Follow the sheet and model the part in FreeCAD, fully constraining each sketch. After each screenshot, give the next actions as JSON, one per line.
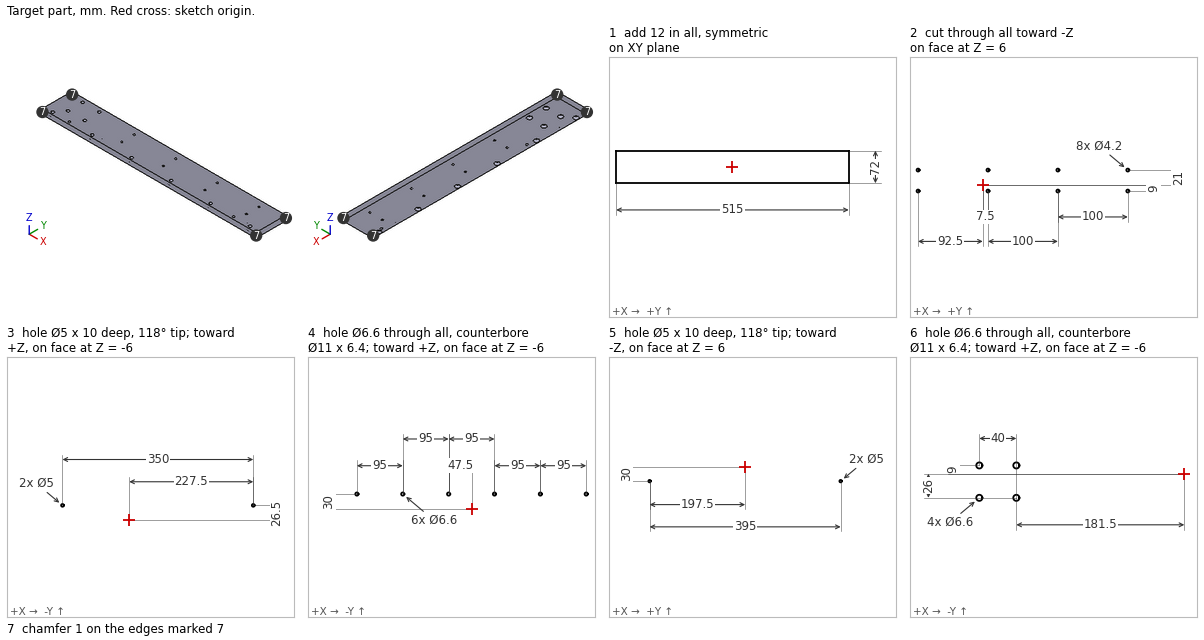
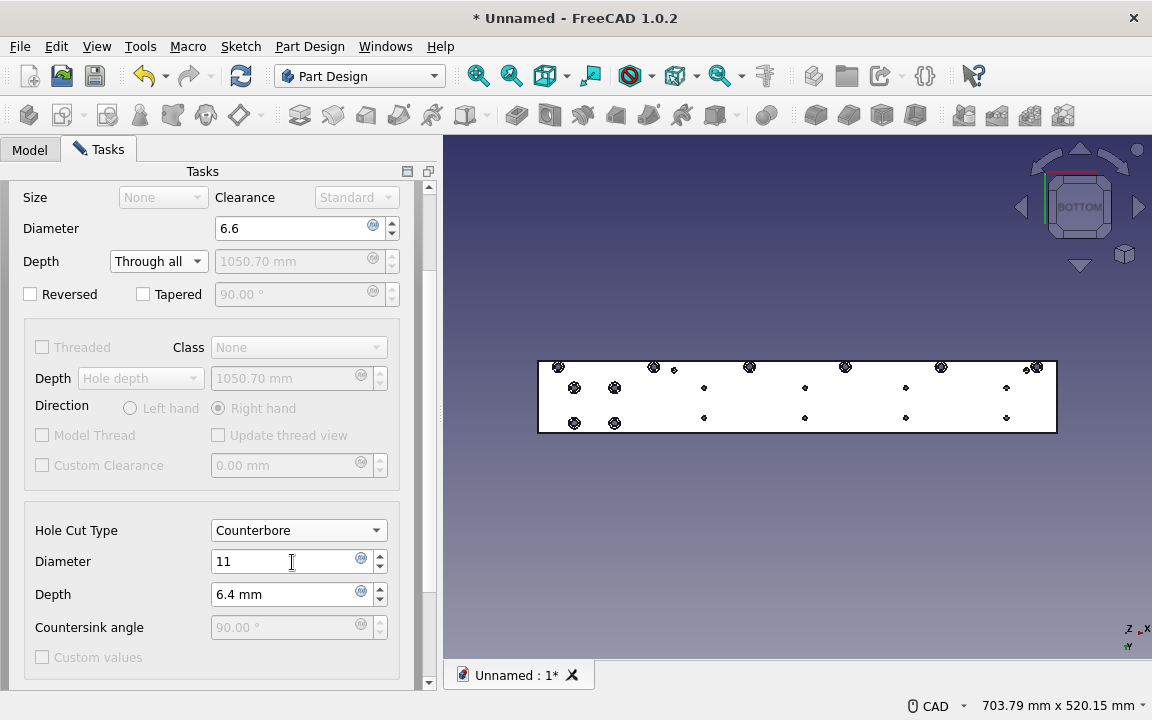
{"action": "scroll", "coordinate": [429, 436], "scroll_direction": "up", "scroll_amount": 3}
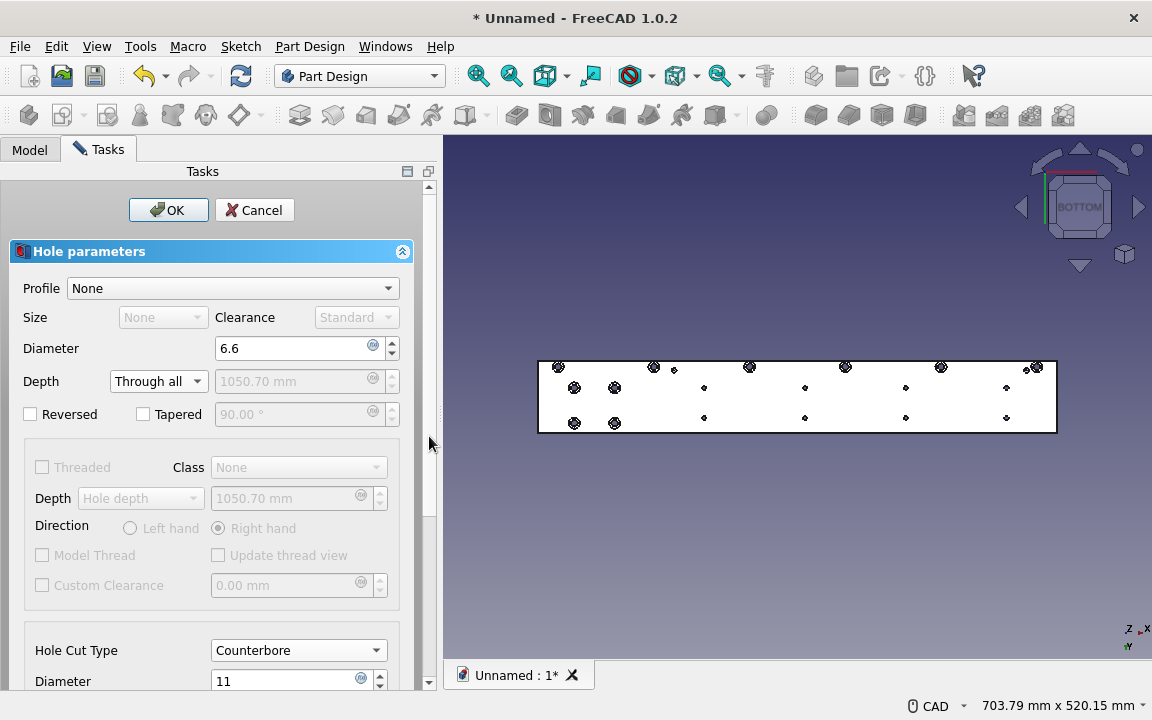
{"action": "left_click", "coordinate": [169, 210]}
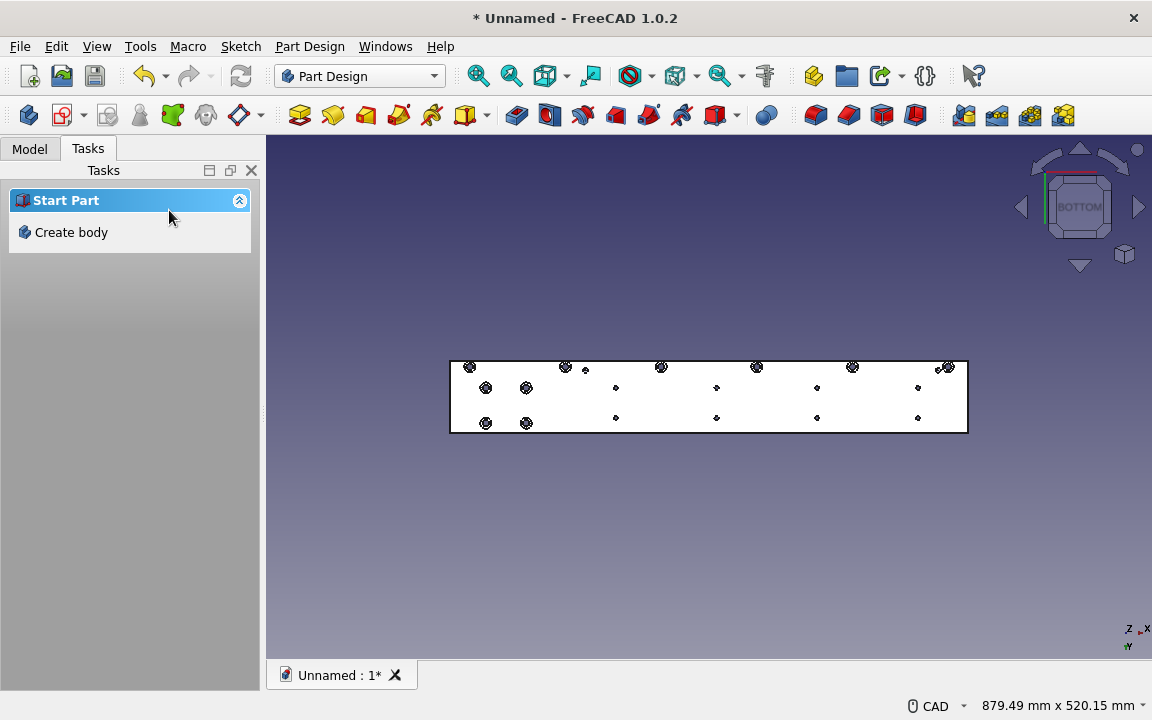
{"action": "scroll", "coordinate": [968, 360], "scroll_direction": "up", "scroll_amount": 6}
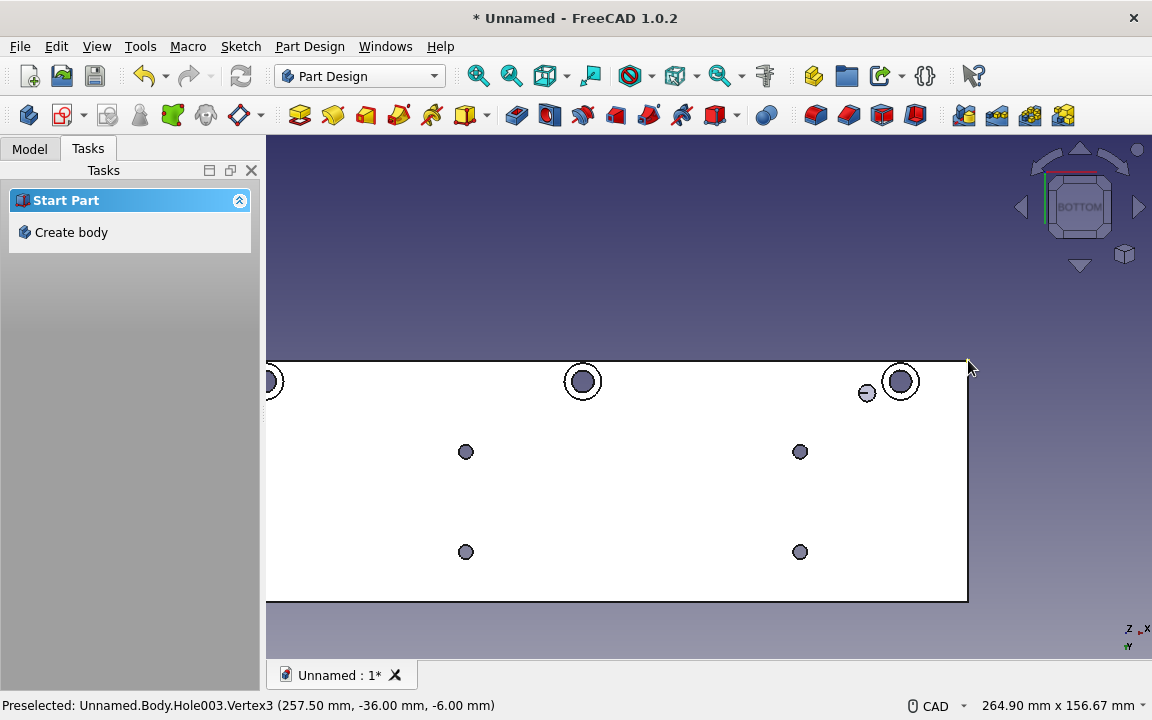
{"action": "left_click", "coordinate": [479, 76]}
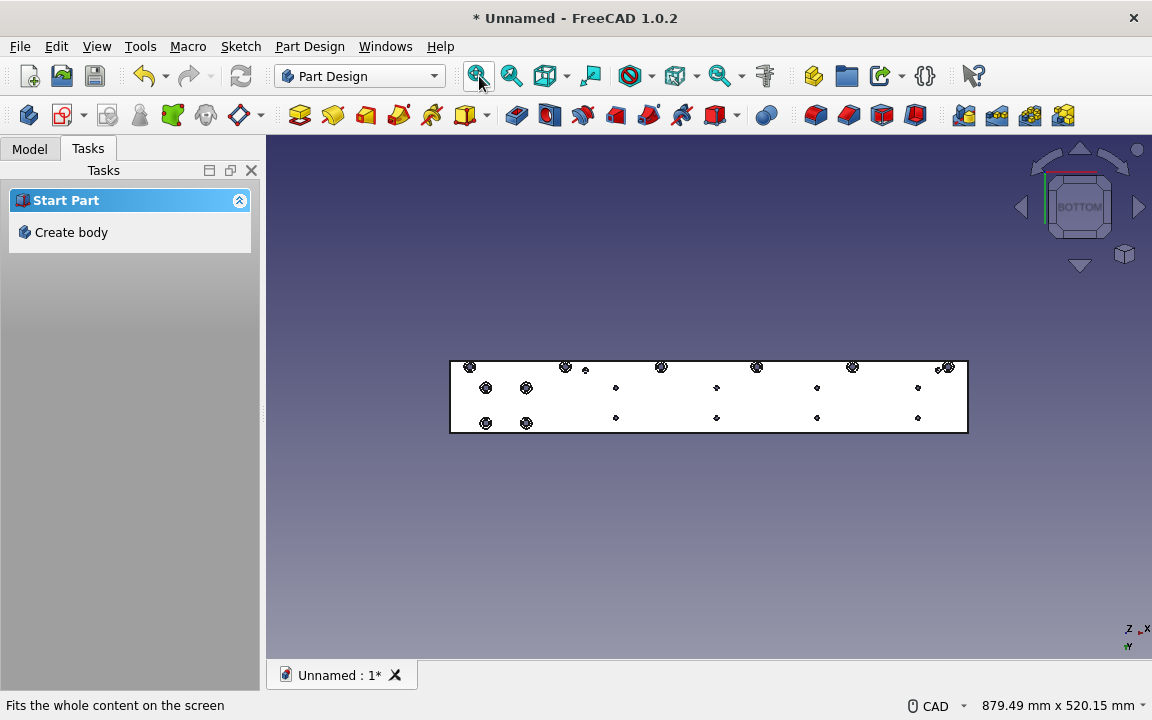
{"action": "key", "text": "0"}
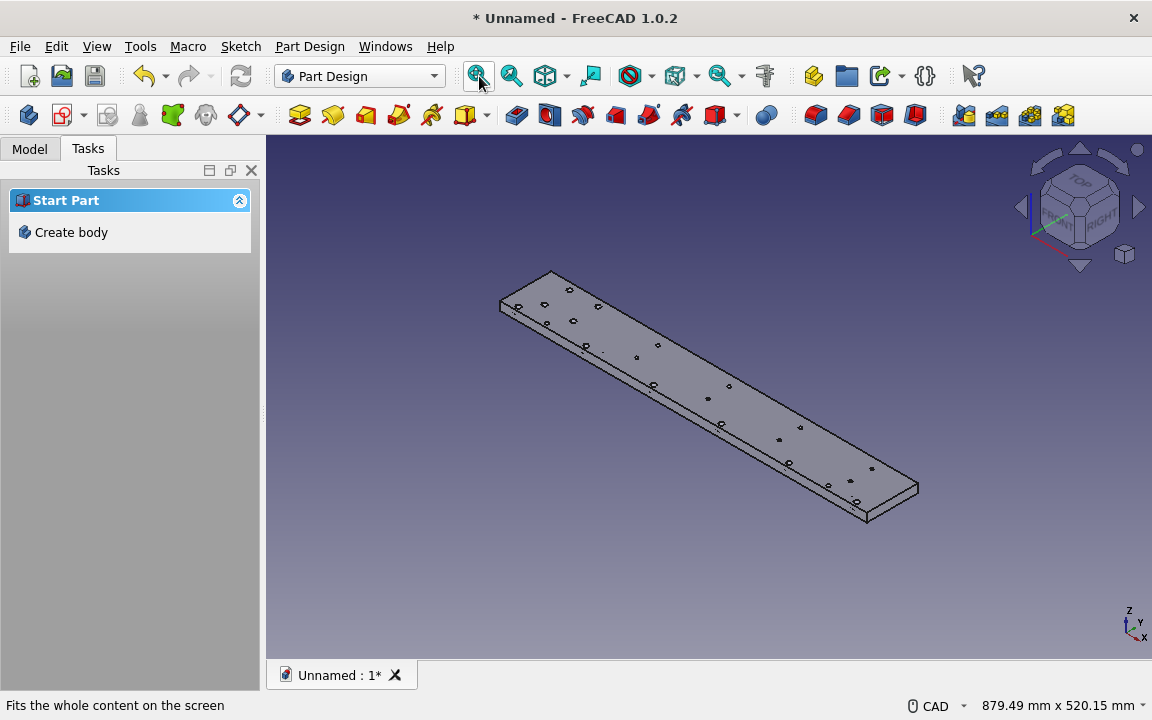
{"action": "left_click", "coordinate": [867, 518]}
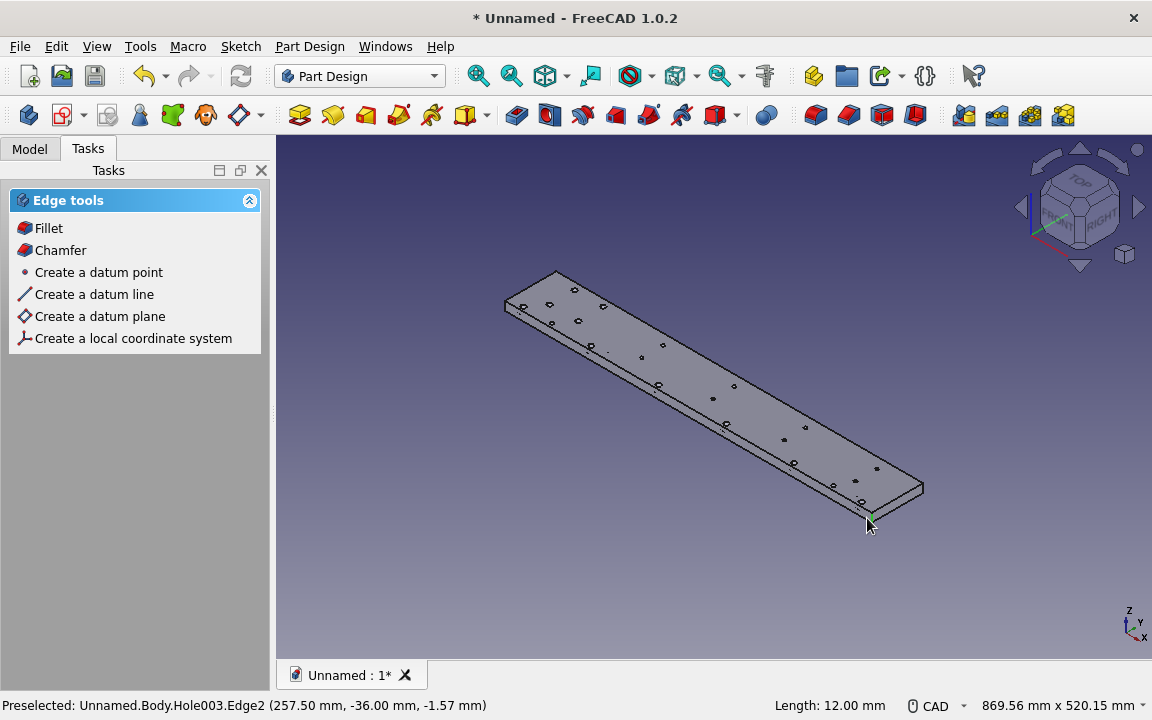
{"action": "scroll", "coordinate": [505, 305], "scroll_direction": "up", "scroll_amount": 6}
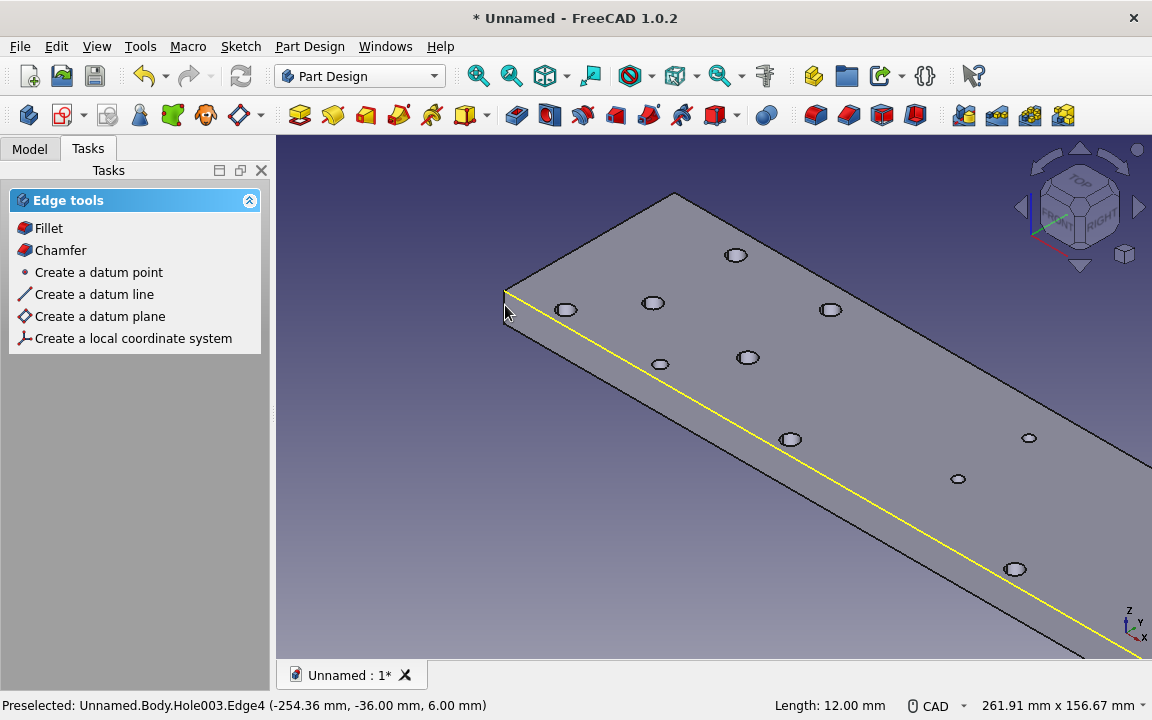
{"action": "left_click", "coordinate": [479, 76]}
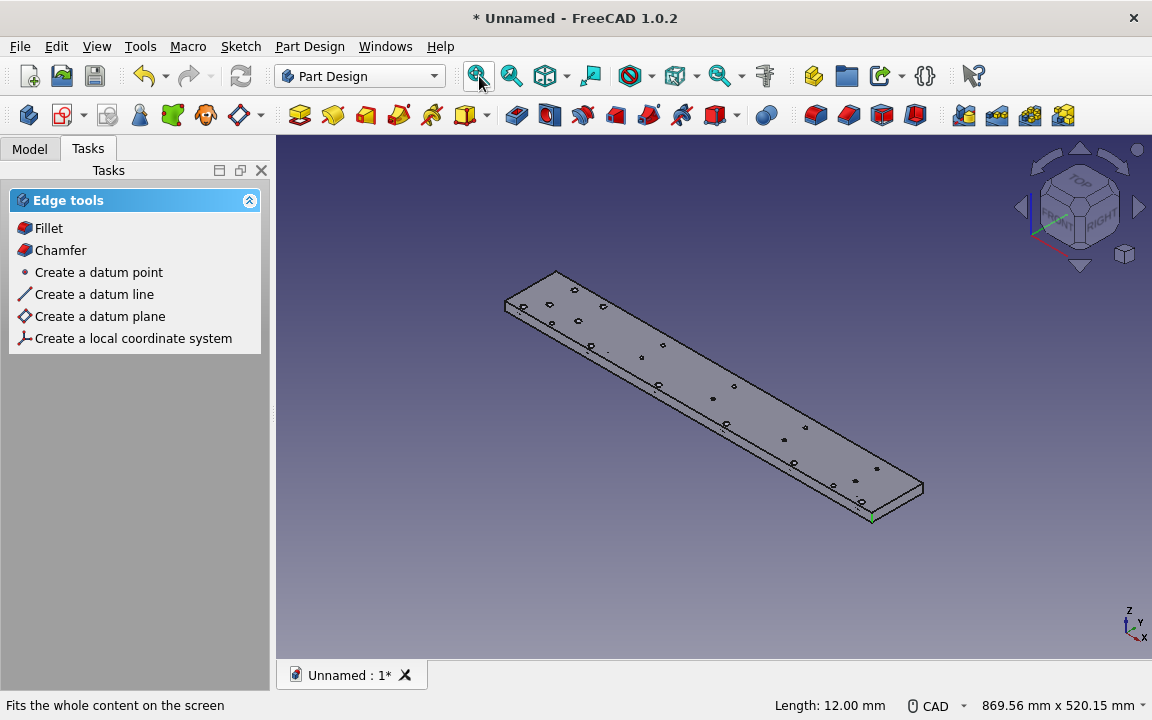
{"action": "key", "text": "2"}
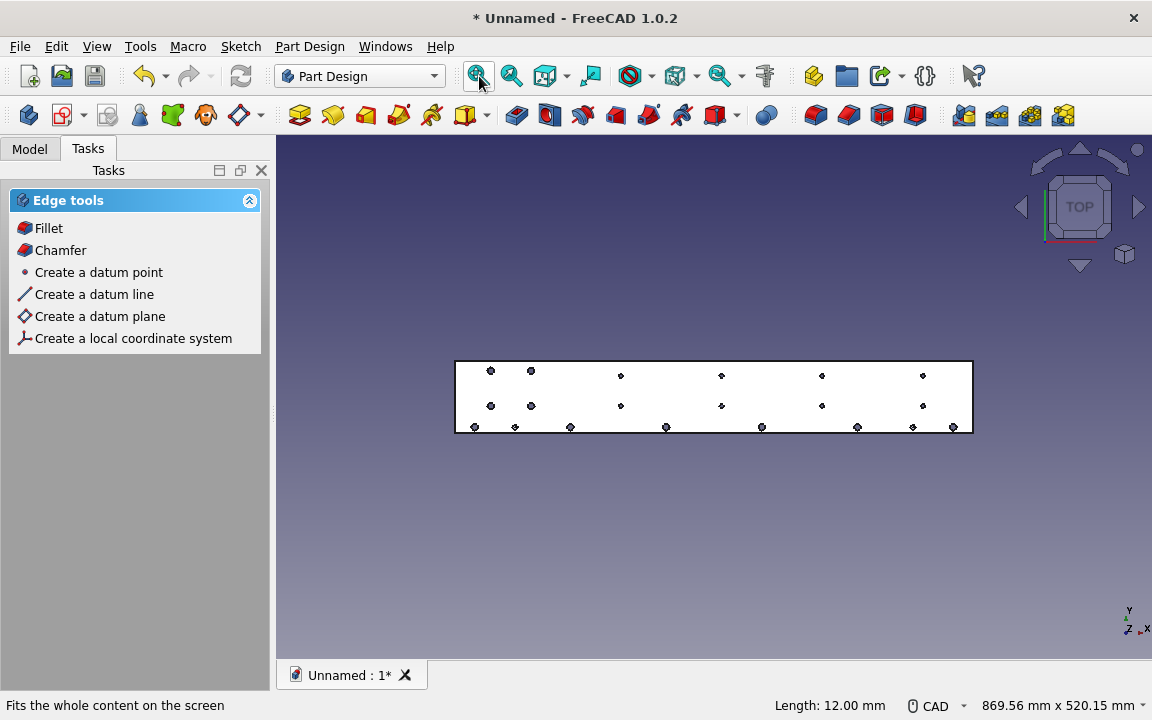
{"action": "scroll", "coordinate": [455, 432], "scroll_direction": "up", "scroll_amount": 6}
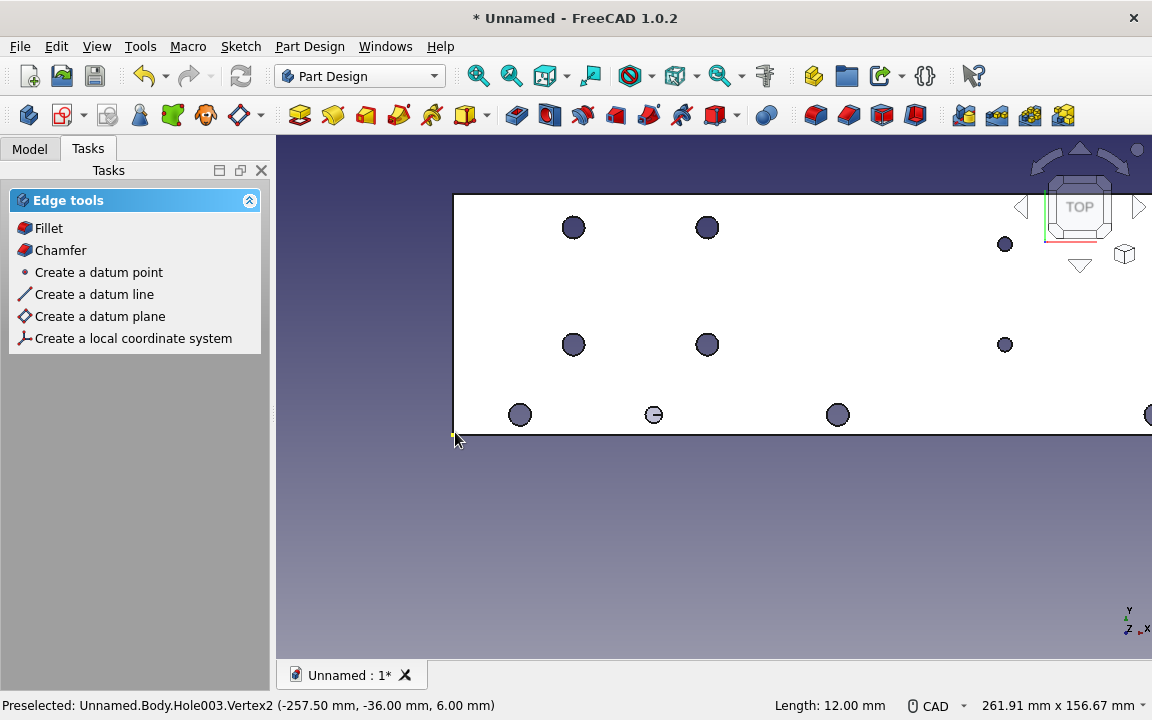
{"action": "left_click", "coordinate": [479, 76]}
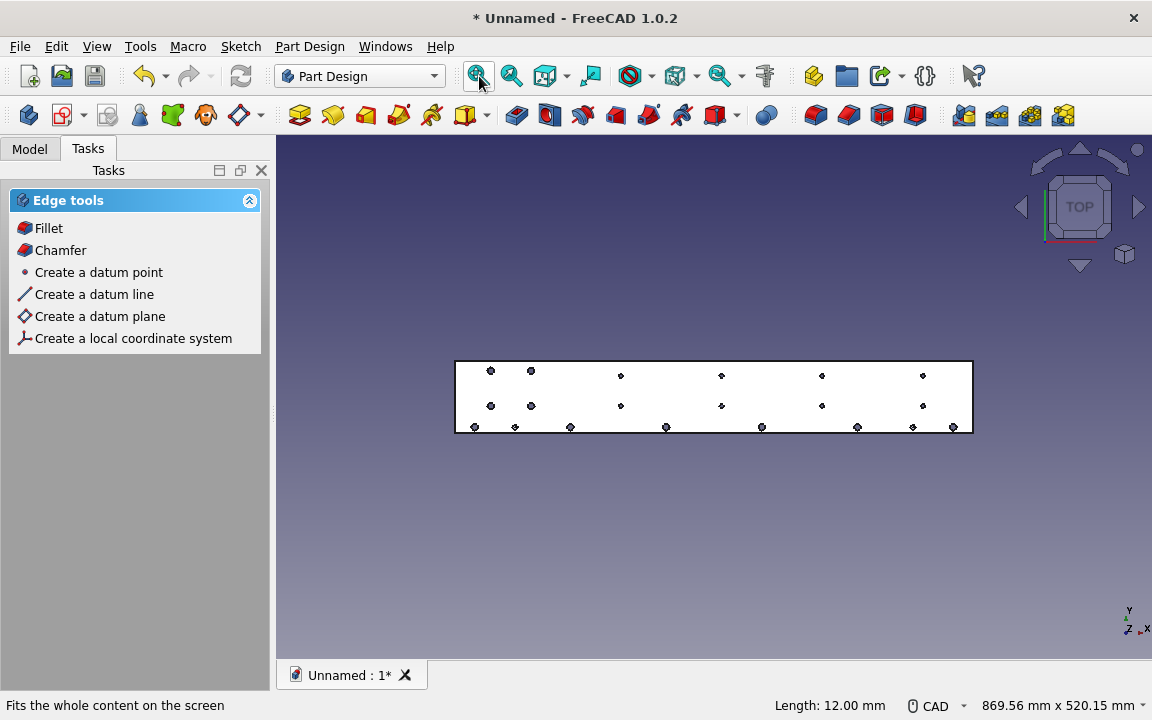
{"action": "key", "text": "1"}